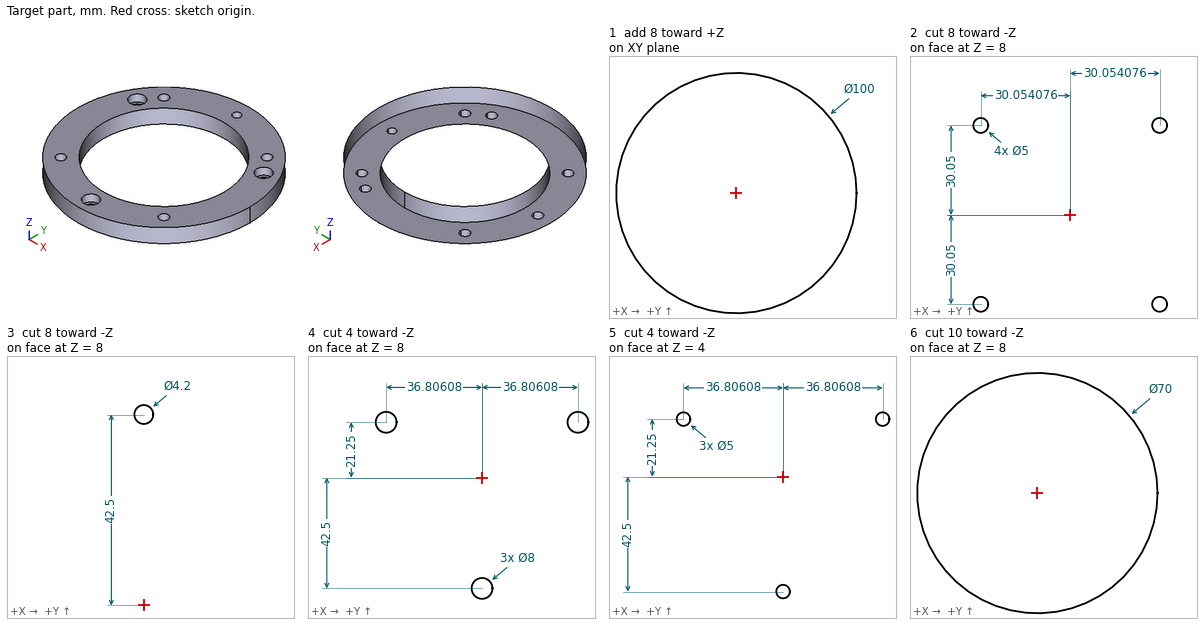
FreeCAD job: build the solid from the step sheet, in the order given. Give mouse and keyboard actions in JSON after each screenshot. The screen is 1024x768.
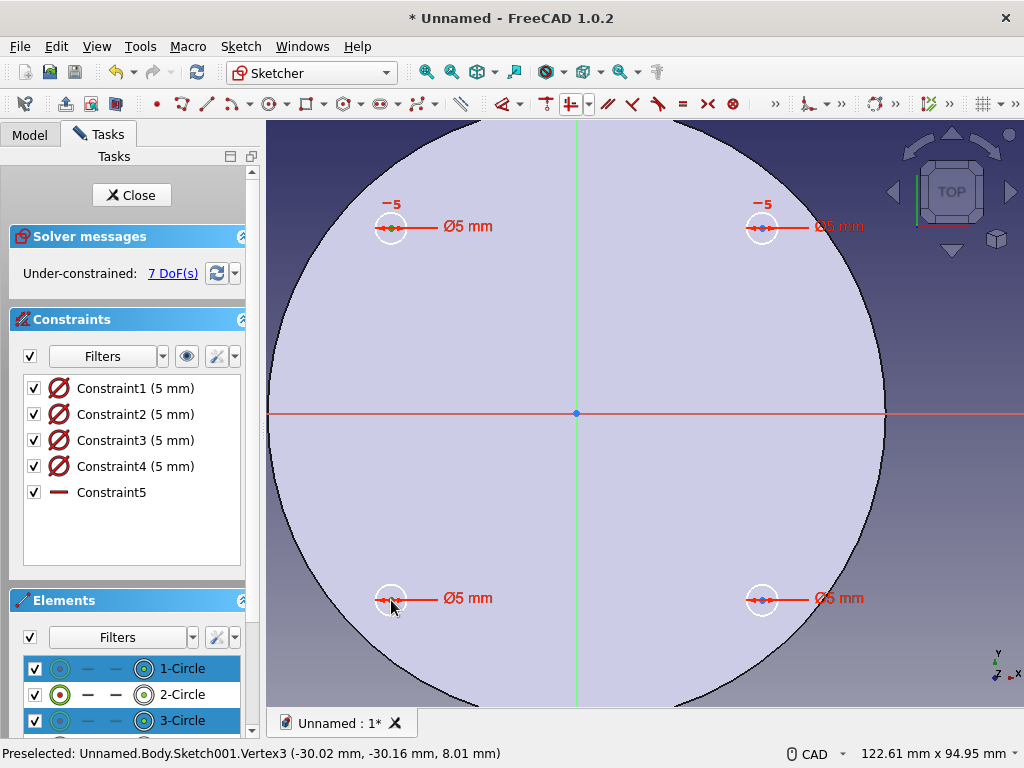
{"action": "key", "text": "v"}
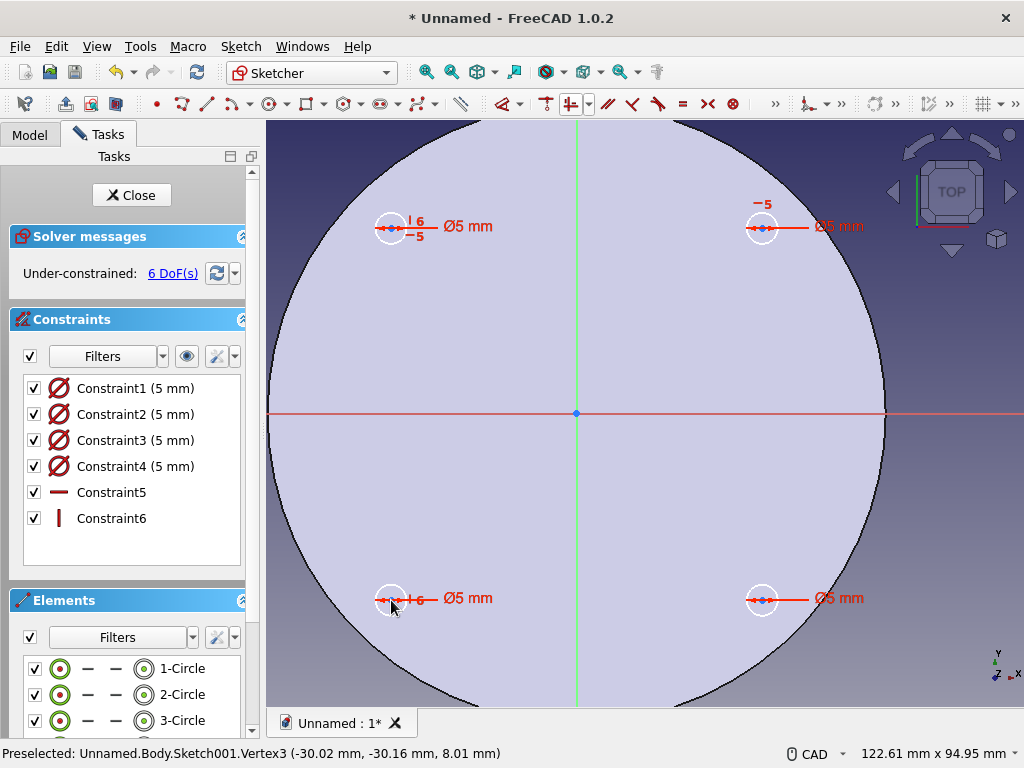
{"action": "left_click", "coordinate": [762, 228]}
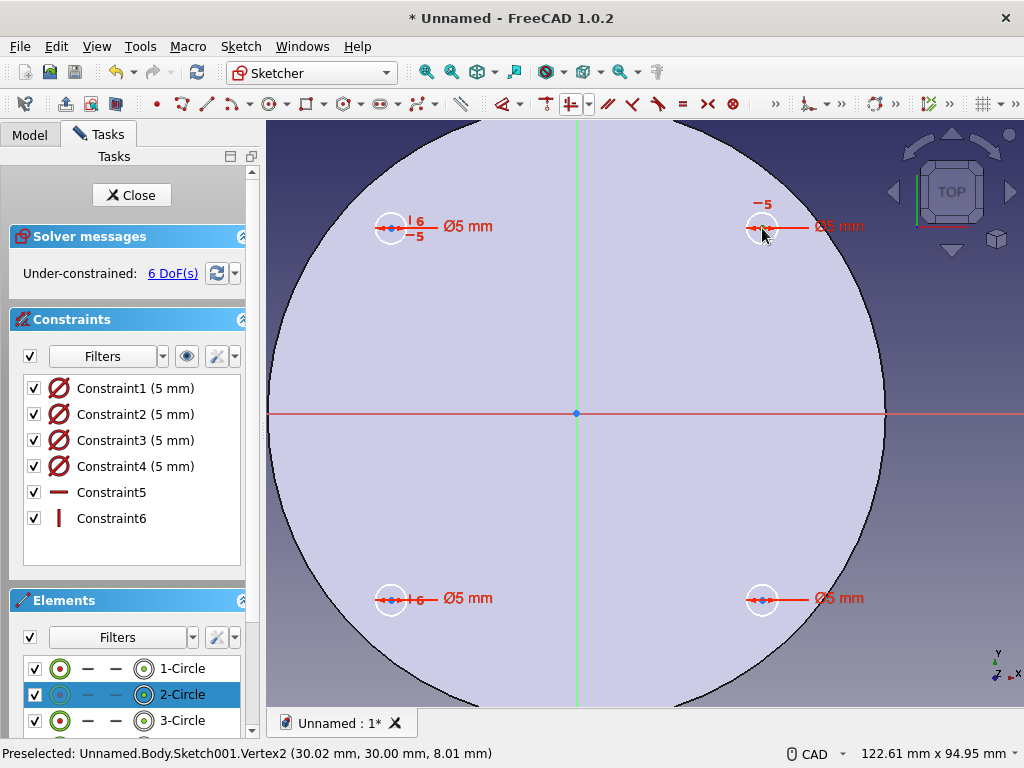
{"action": "left_click", "coordinate": [762, 600]}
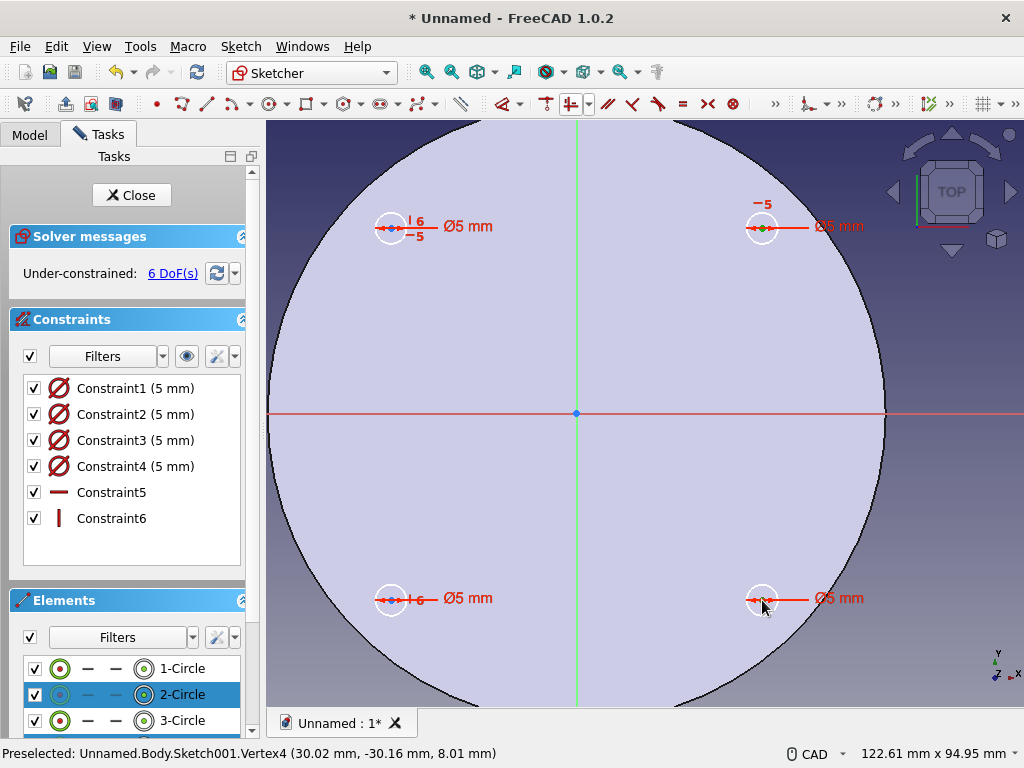
{"action": "left_click", "coordinate": [588, 104]}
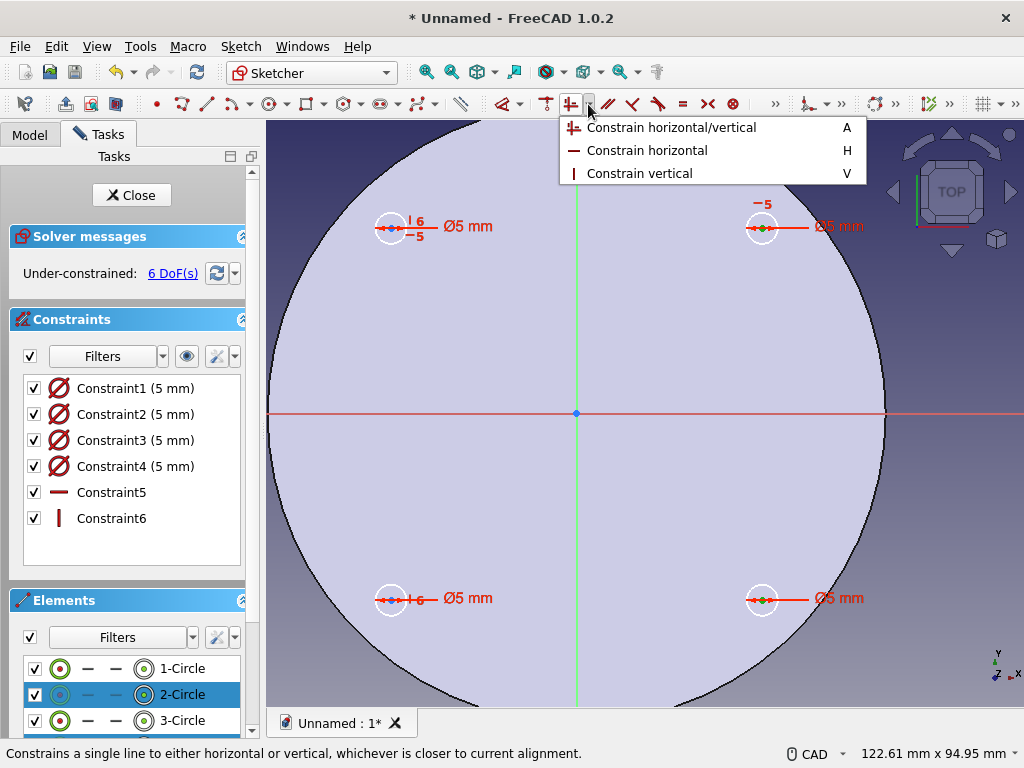
{"action": "left_click", "coordinate": [713, 174]}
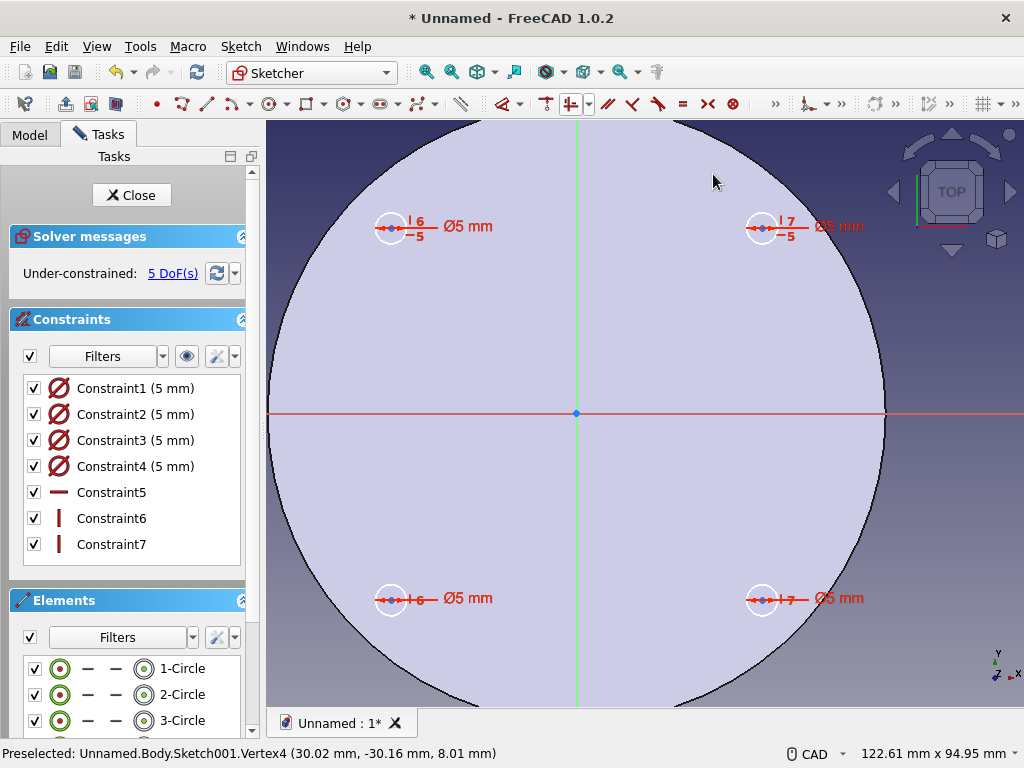
{"action": "left_click", "coordinate": [391, 600]}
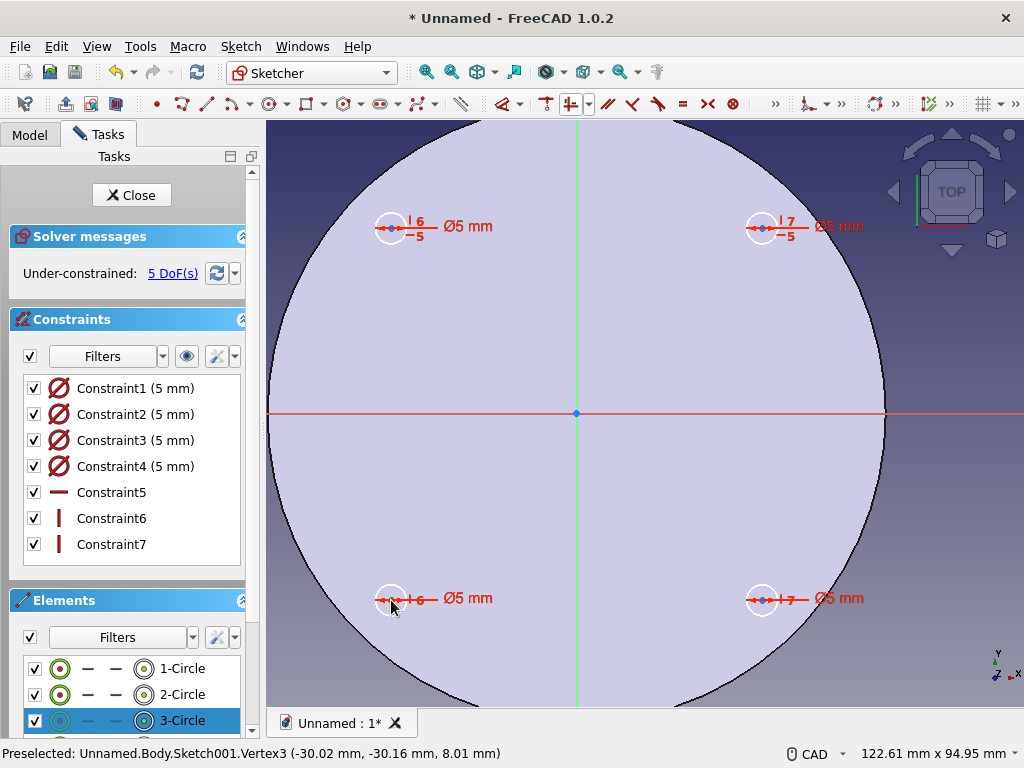
{"action": "left_click", "coordinate": [762, 600]}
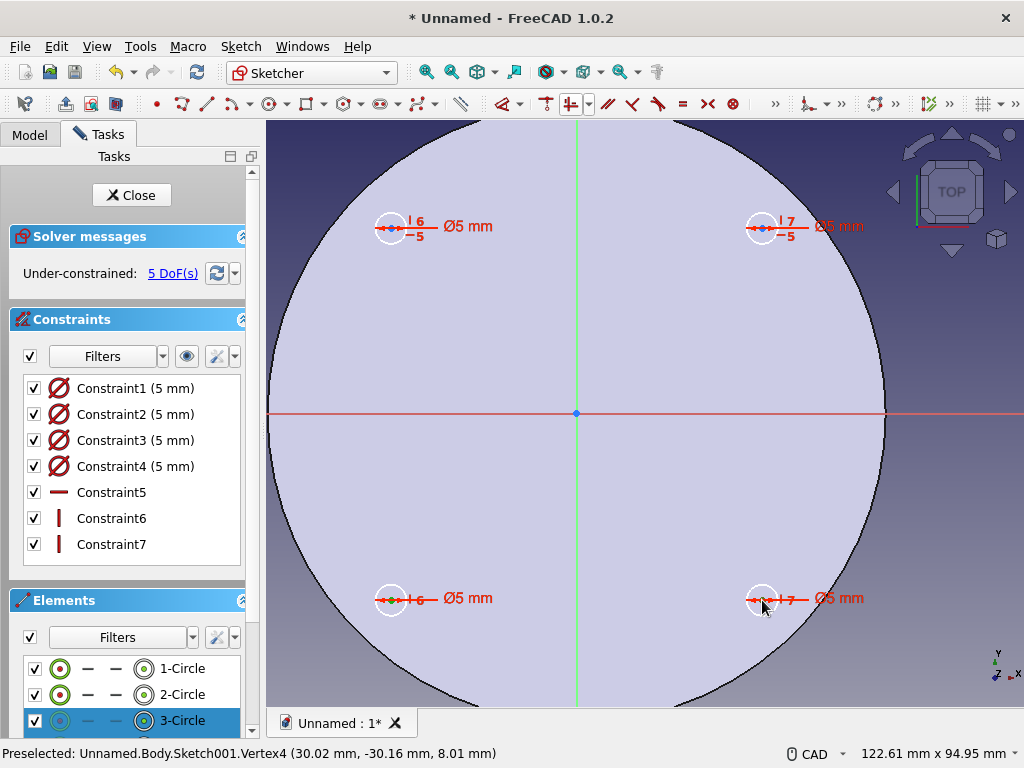
{"action": "left_click", "coordinate": [588, 104]}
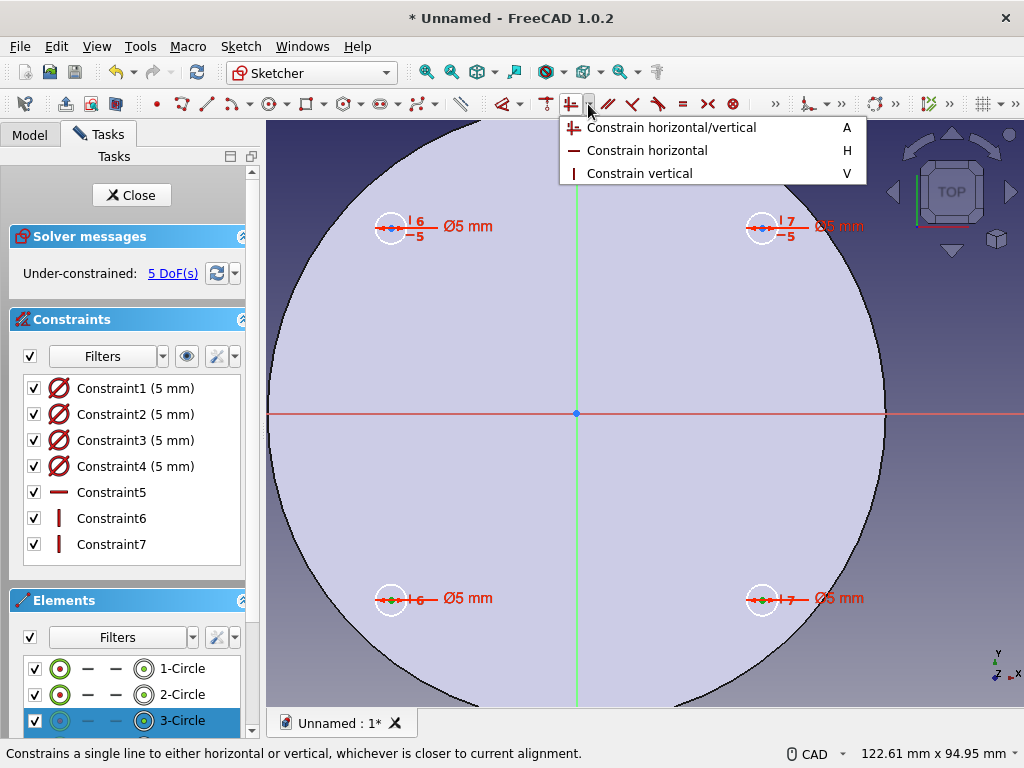
{"action": "left_click", "coordinate": [713, 150]}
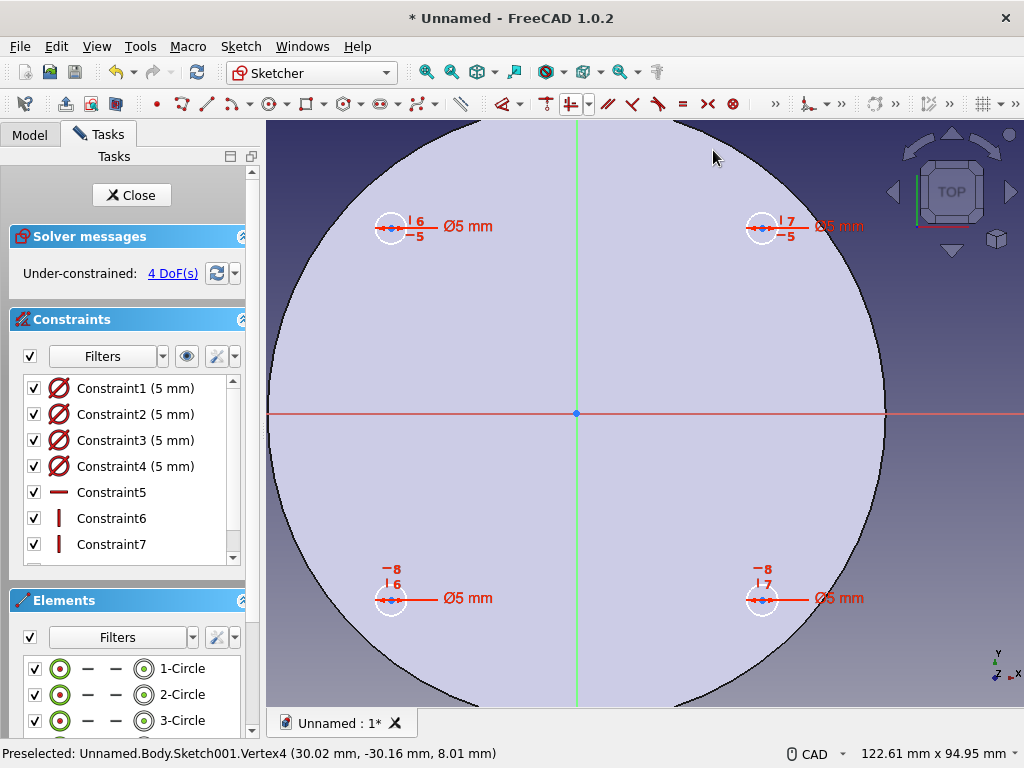
{"action": "left_click", "coordinate": [502, 104]}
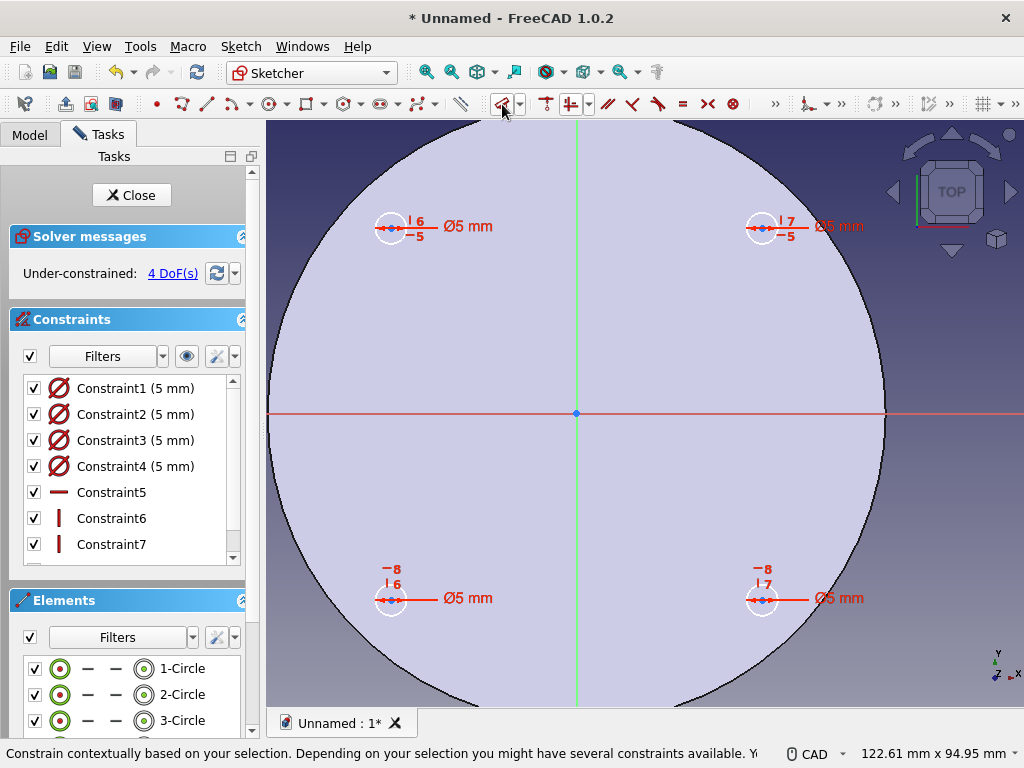
{"action": "left_click", "coordinate": [391, 228]}
{"action": "left_click", "coordinate": [357, 321]}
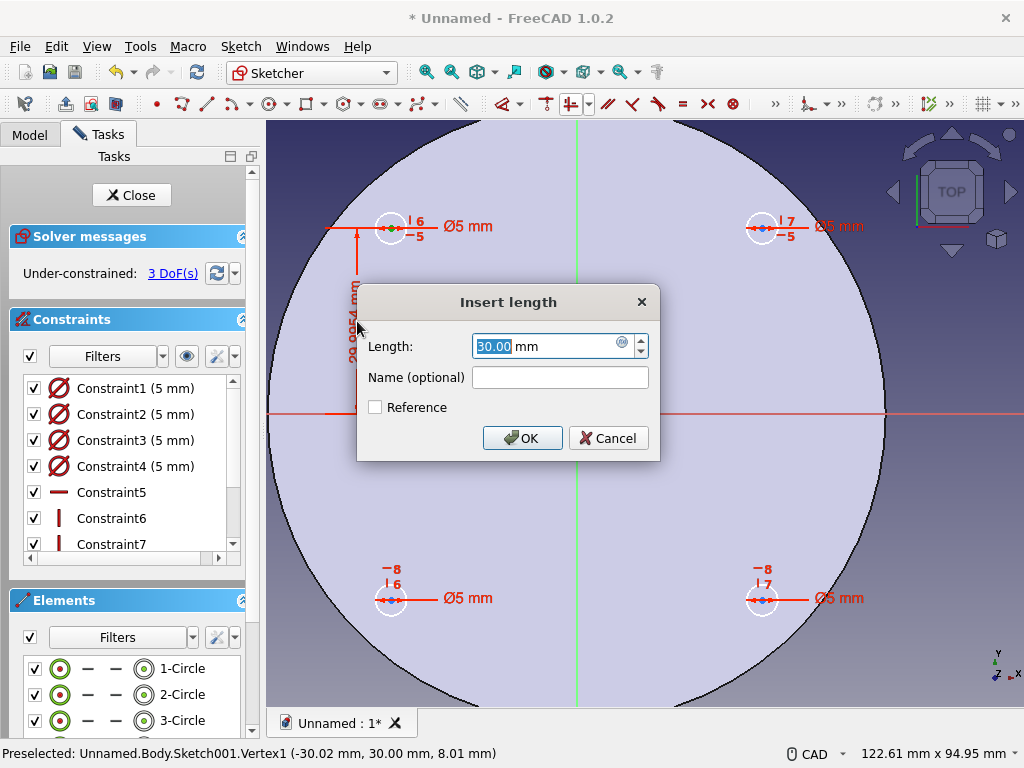
{"action": "type", "text": "30.05"}
{"action": "key", "text": "Return"}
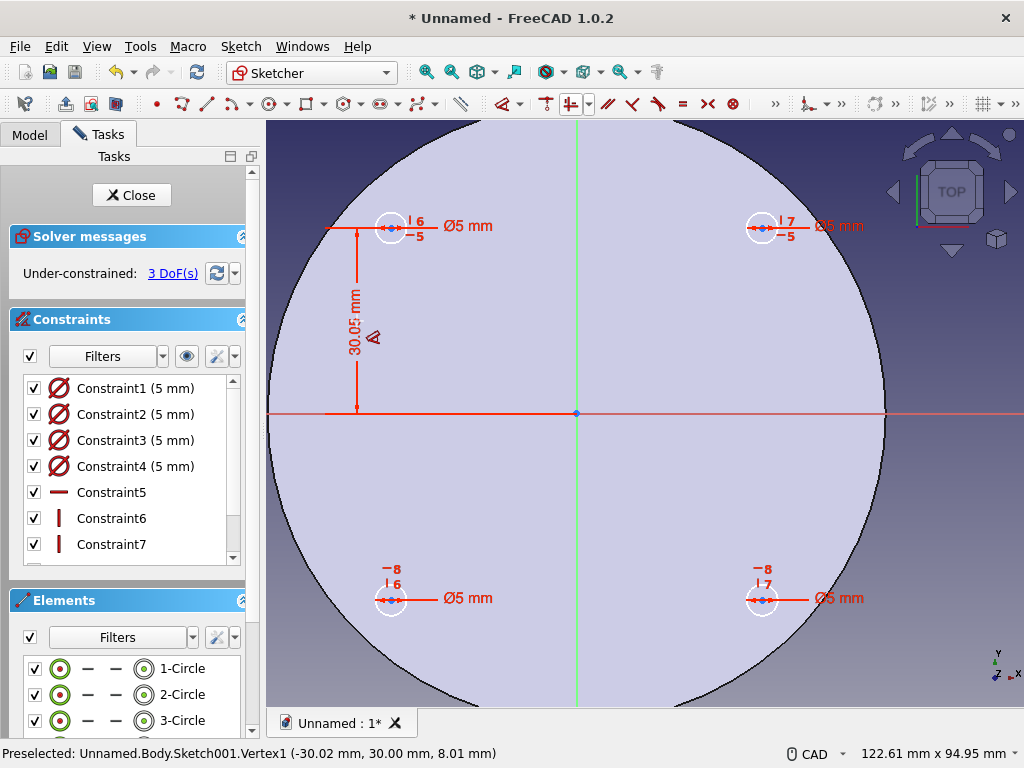
{"action": "left_click", "coordinate": [391, 600]}
{"action": "left_click", "coordinate": [357, 507]}